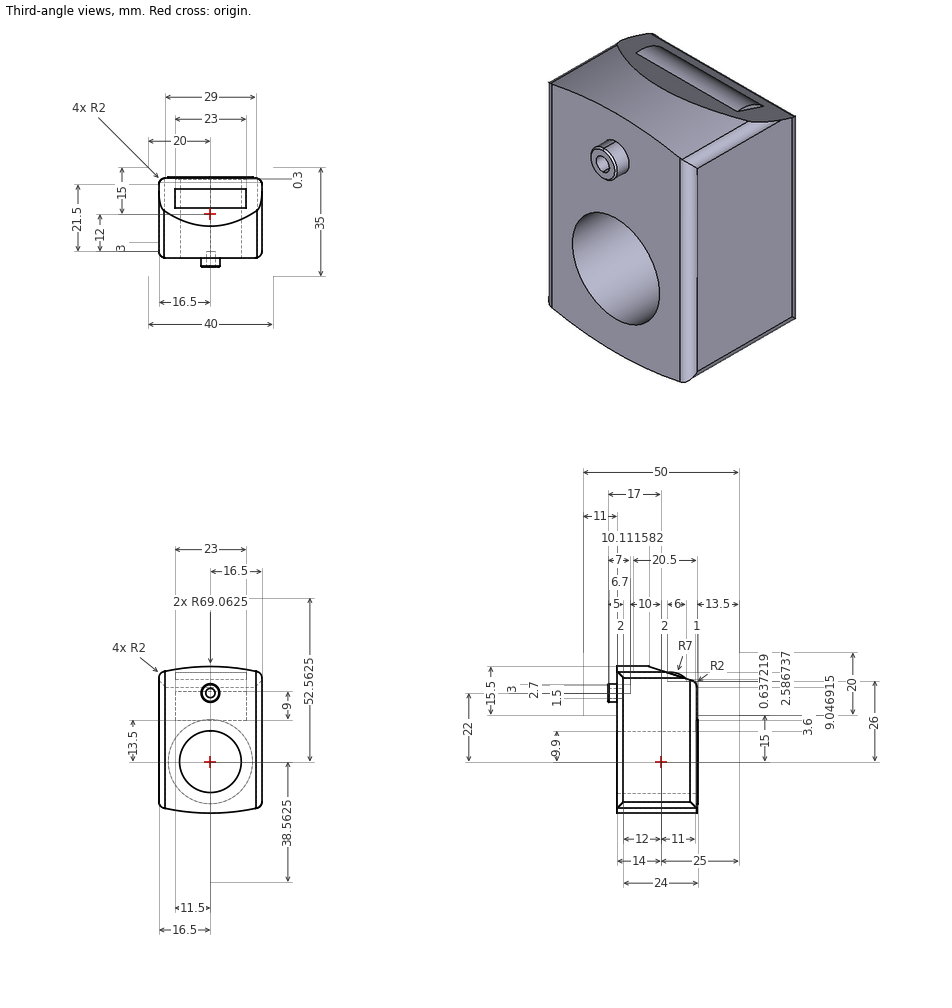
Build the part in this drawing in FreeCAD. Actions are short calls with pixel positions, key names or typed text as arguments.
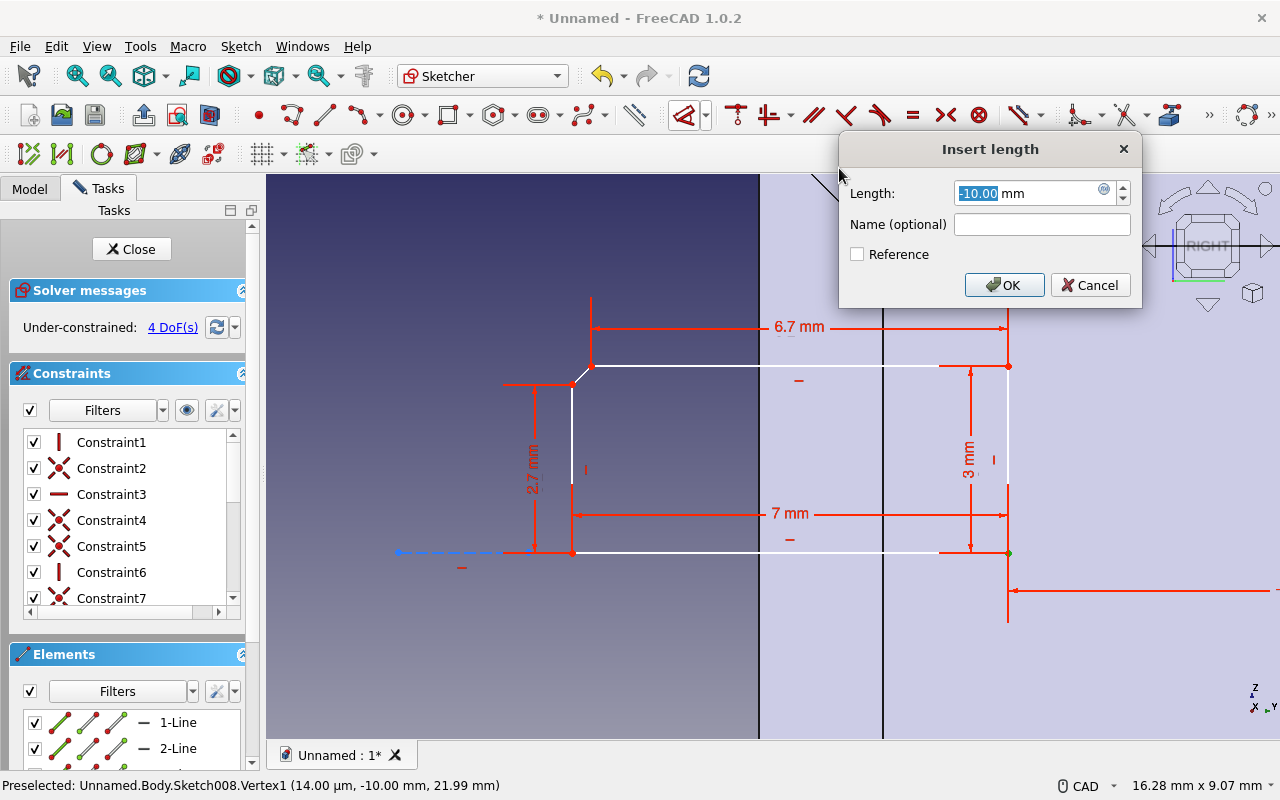
text(-10)
key(Return)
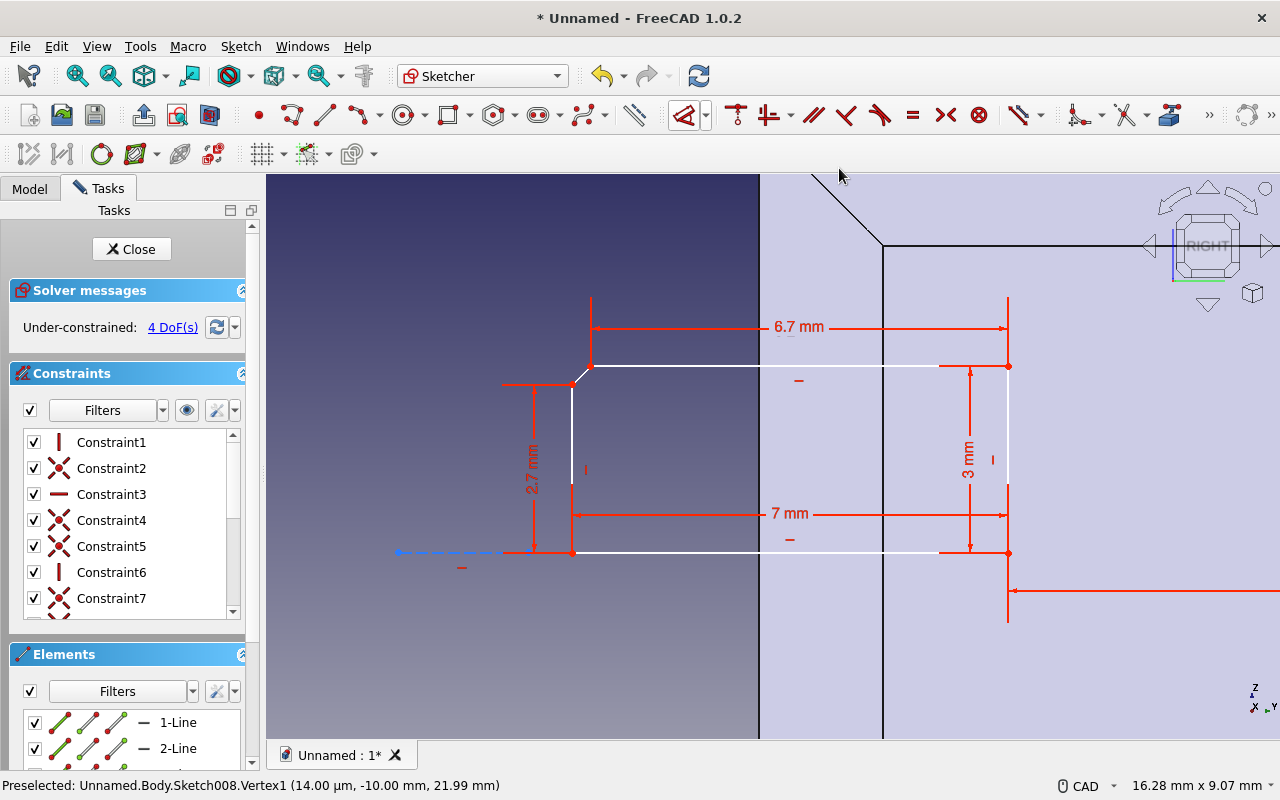
click(1008, 553)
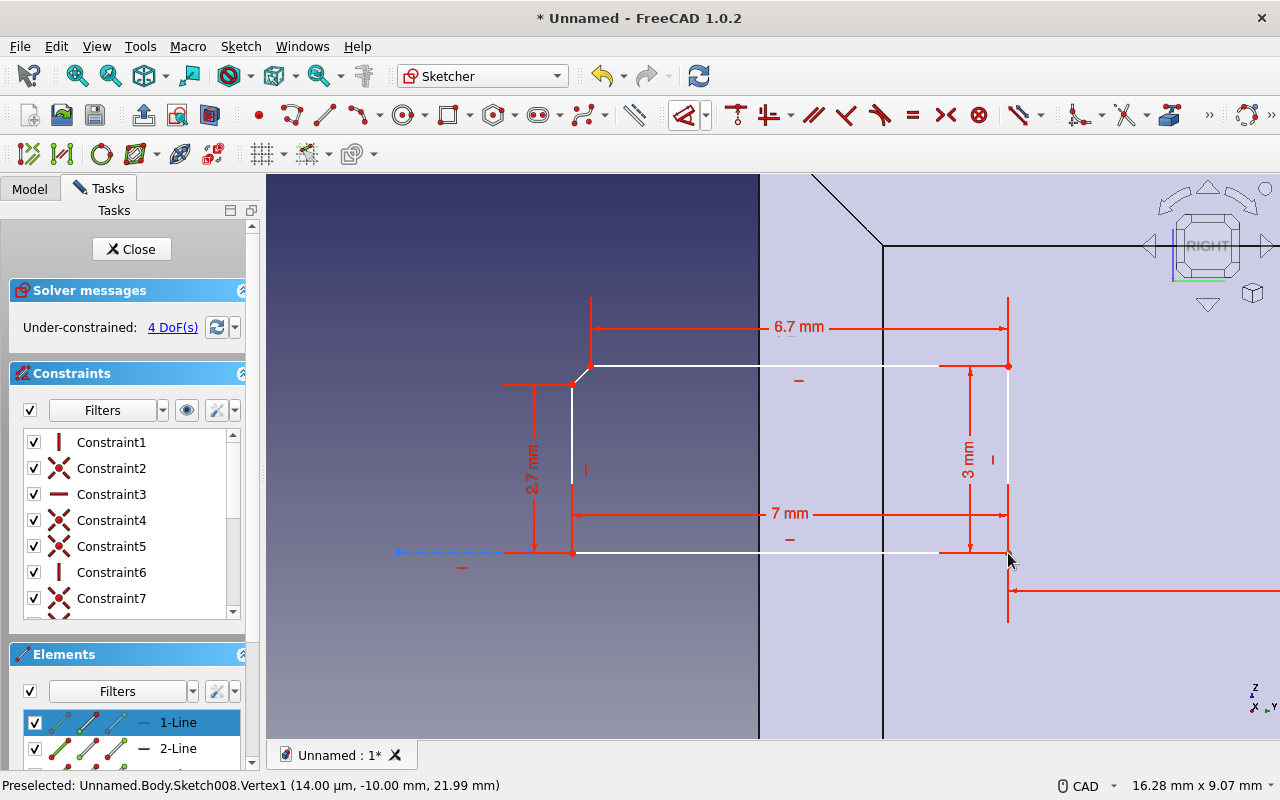
key(i)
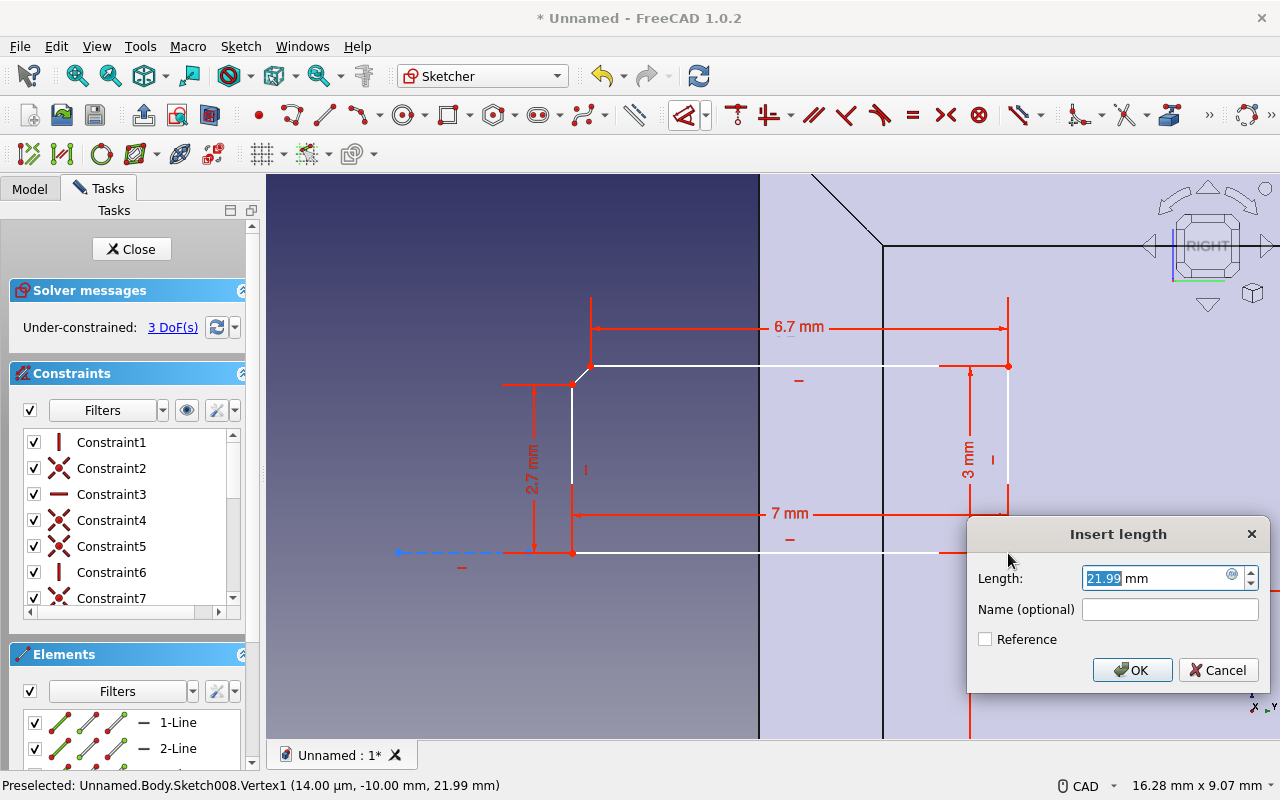
text(22)
key(Return)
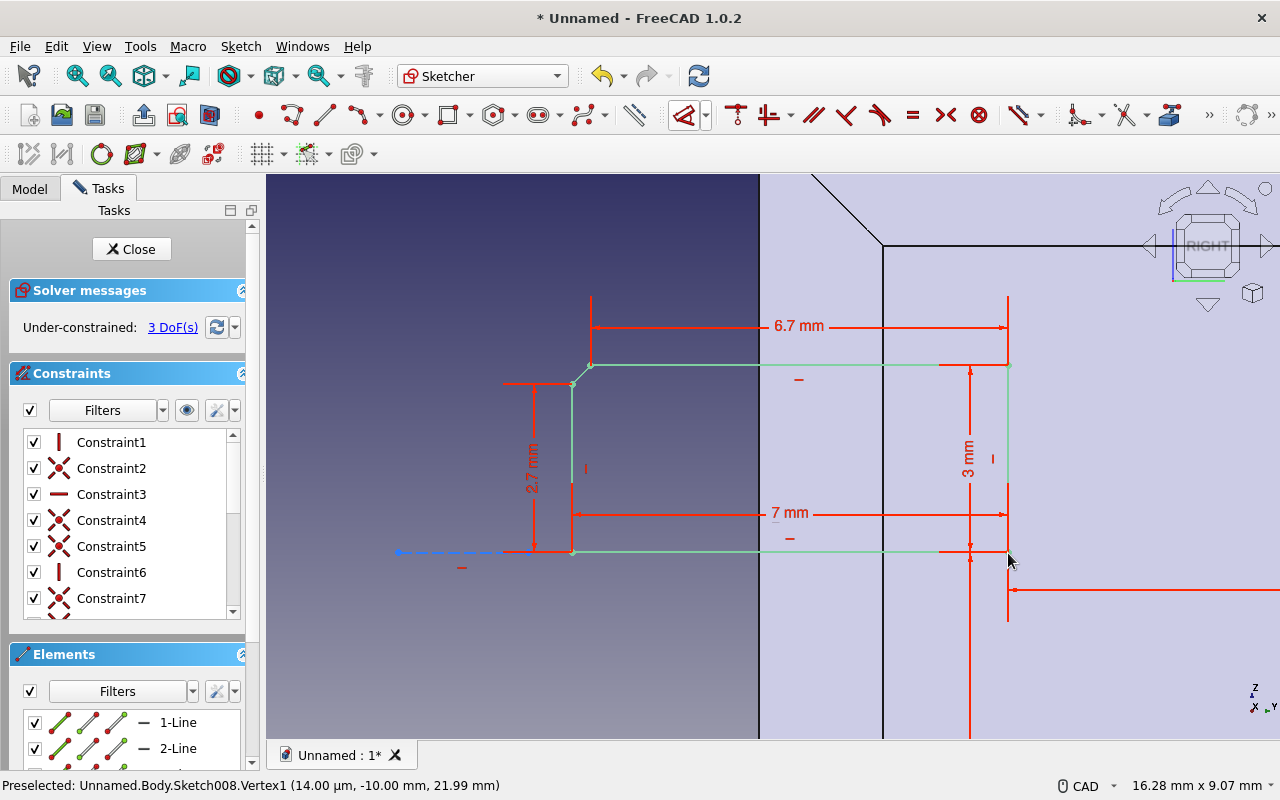
click(528, 553)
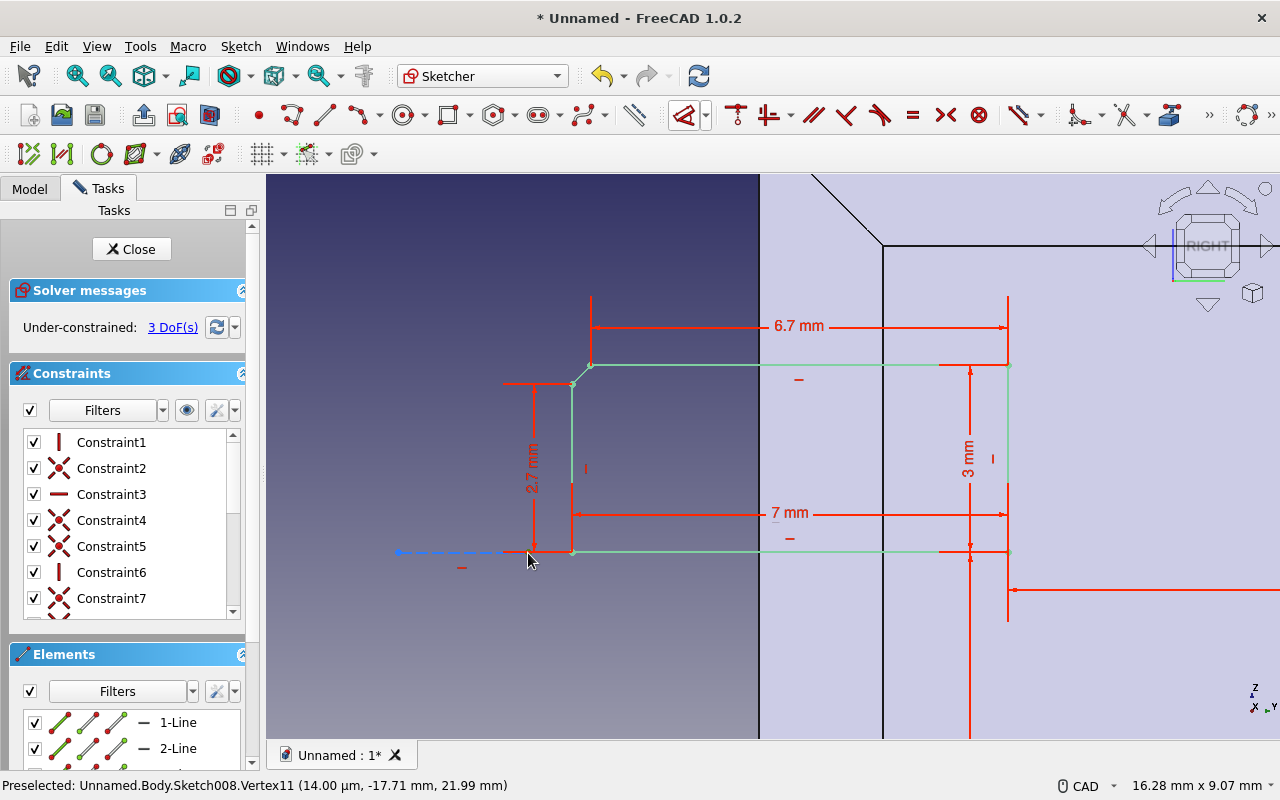
click(706, 116)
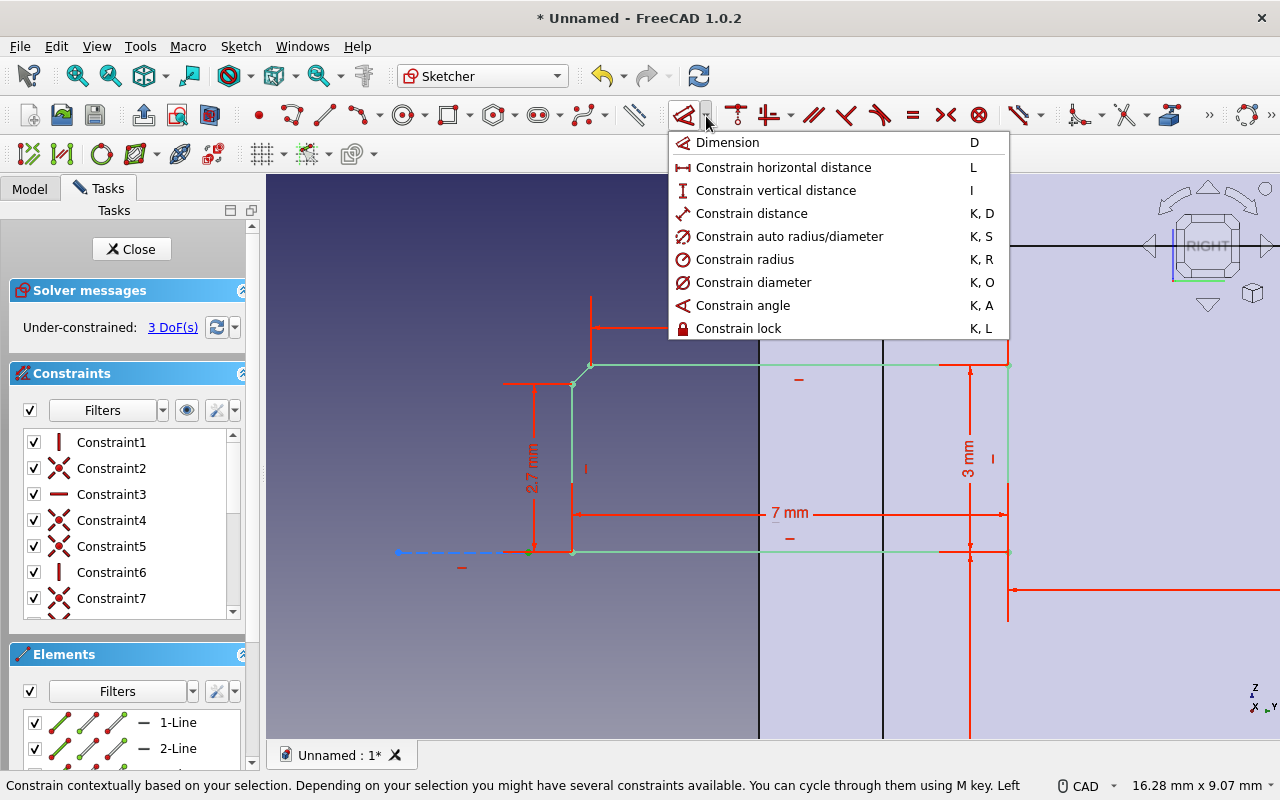
click(839, 190)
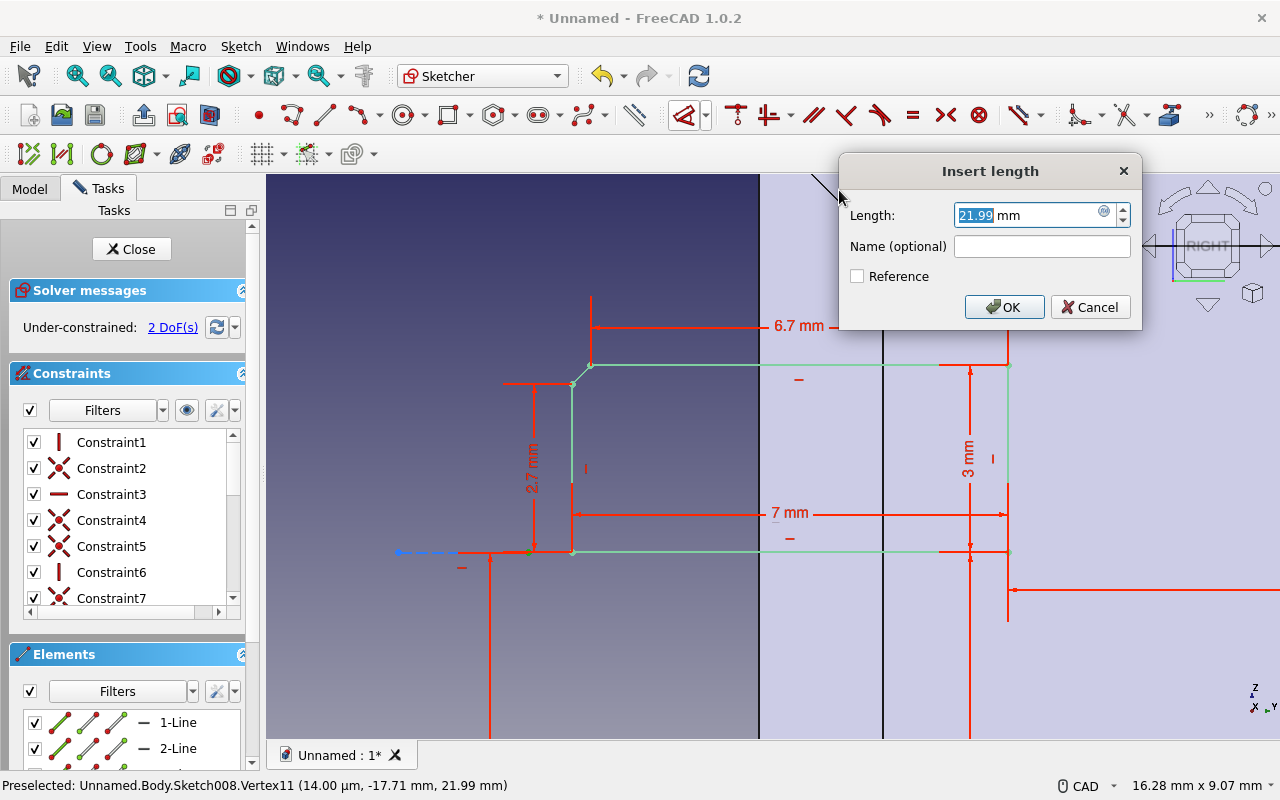
text(22)
key(Return)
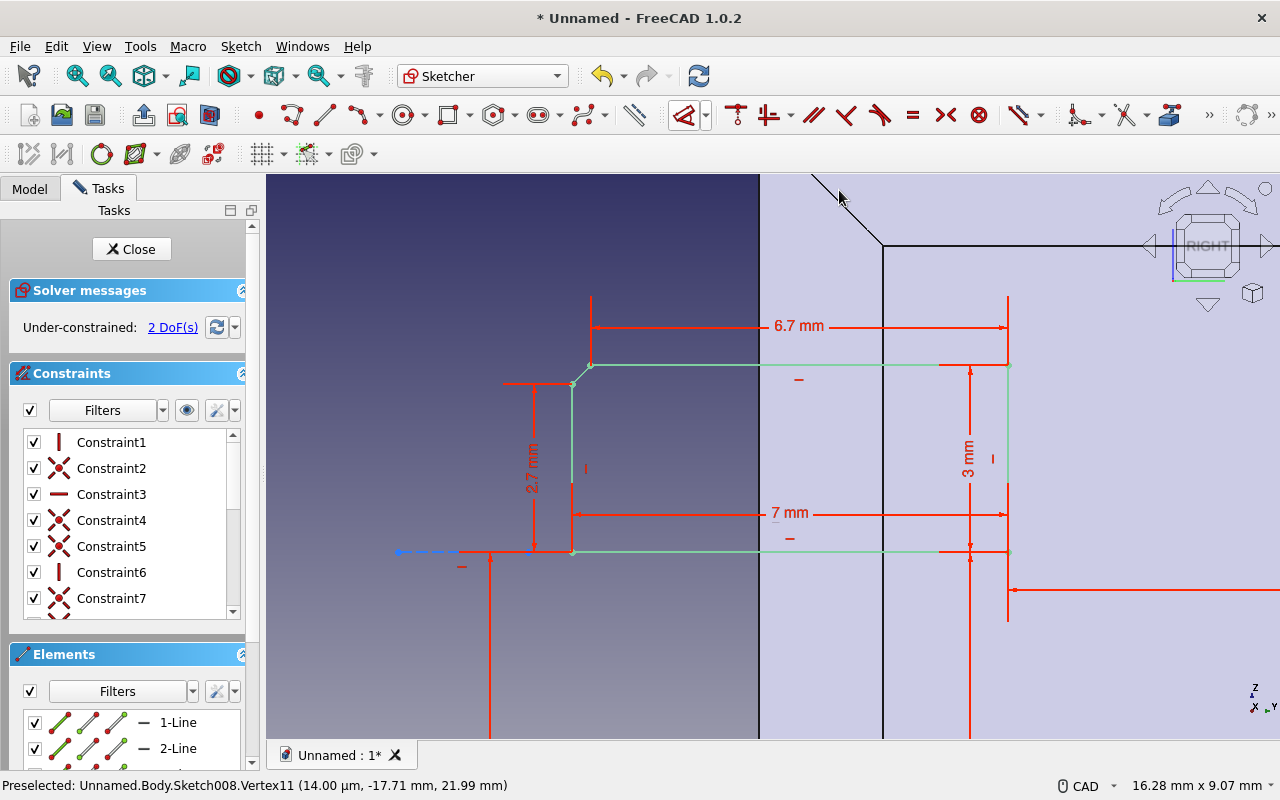
click(132, 249)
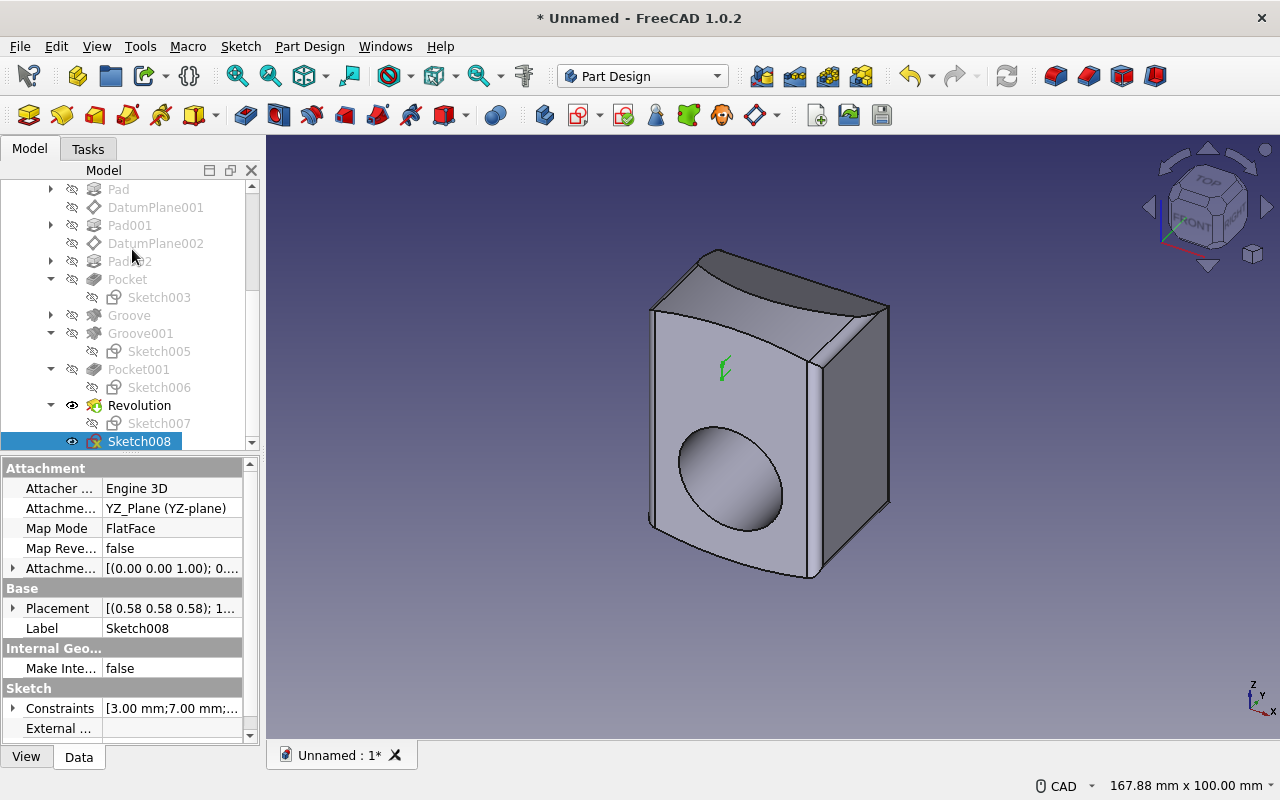
click(62, 116)